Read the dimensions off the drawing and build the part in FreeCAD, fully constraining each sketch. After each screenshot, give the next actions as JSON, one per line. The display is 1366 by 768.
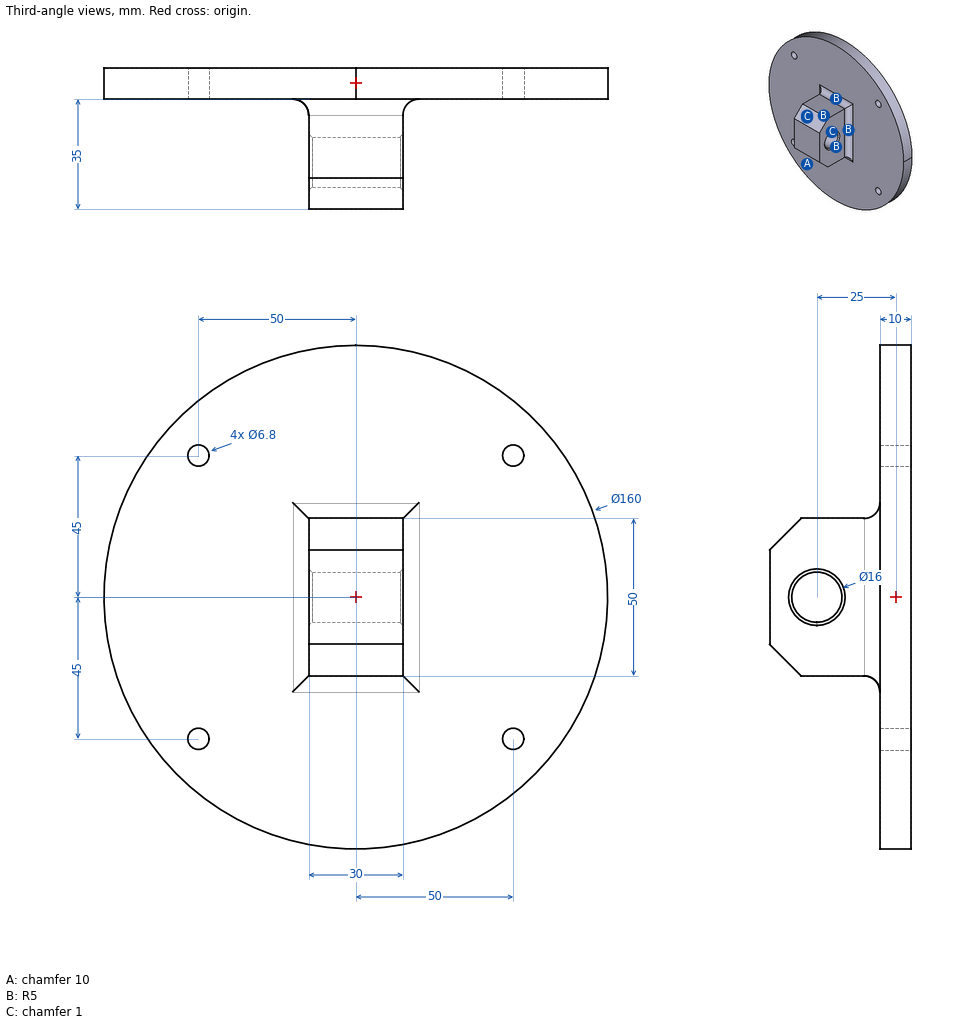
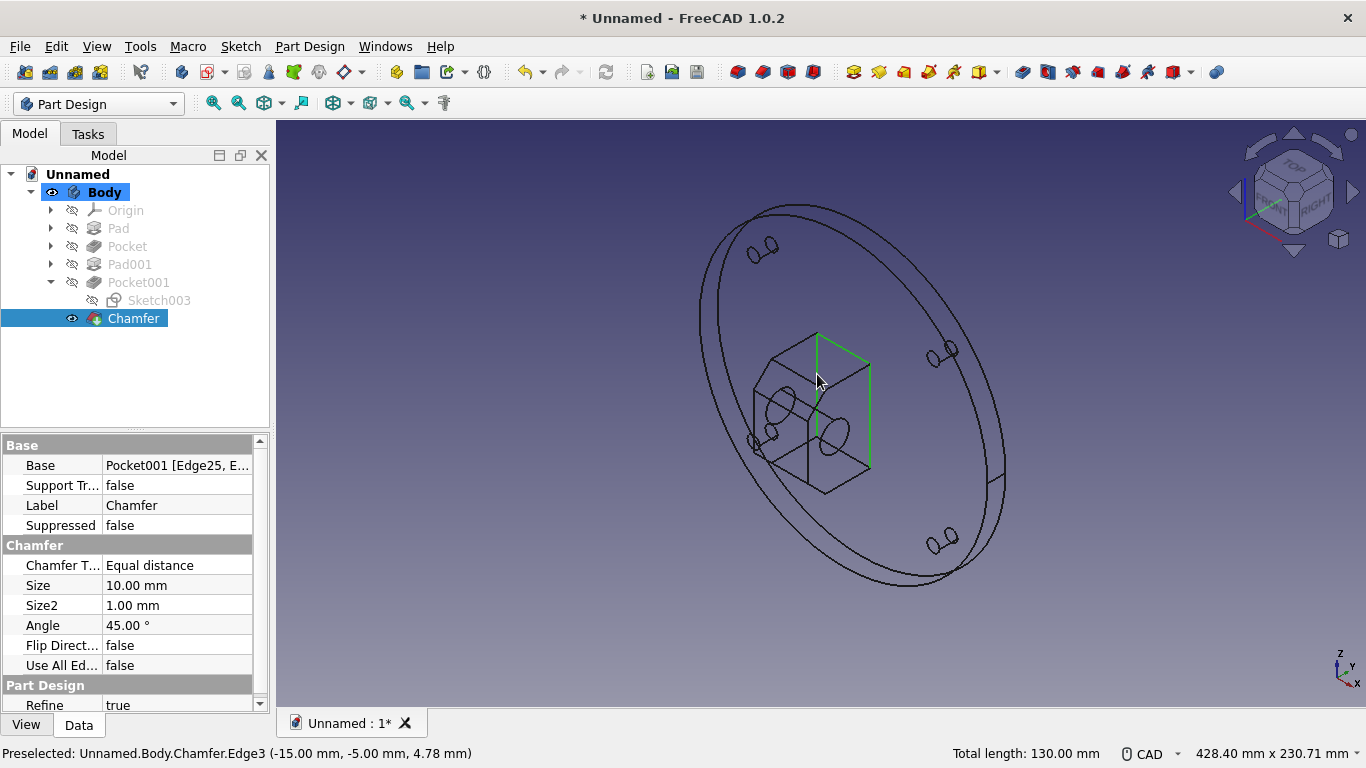
{"action": "left_click", "coordinate": [849, 455], "text": "ctrl"}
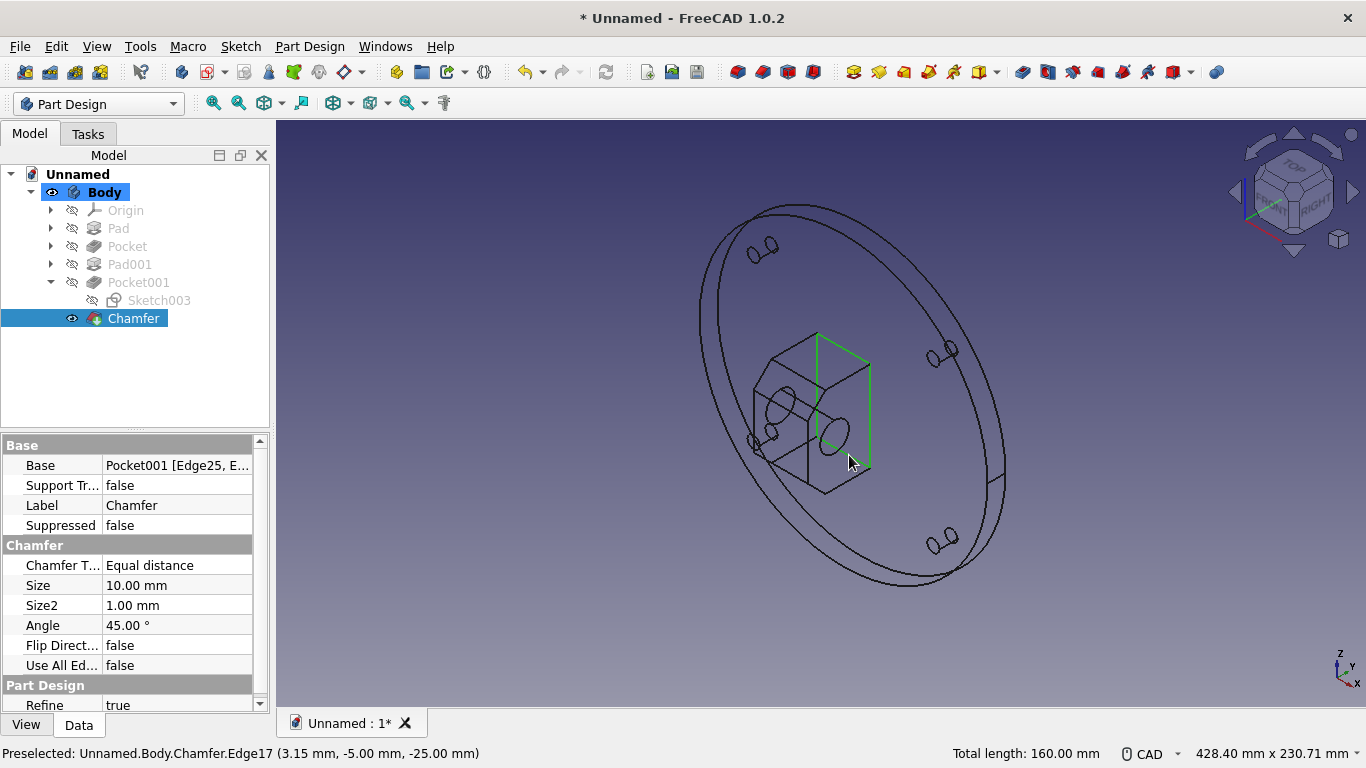
{"action": "key", "text": "v 1"}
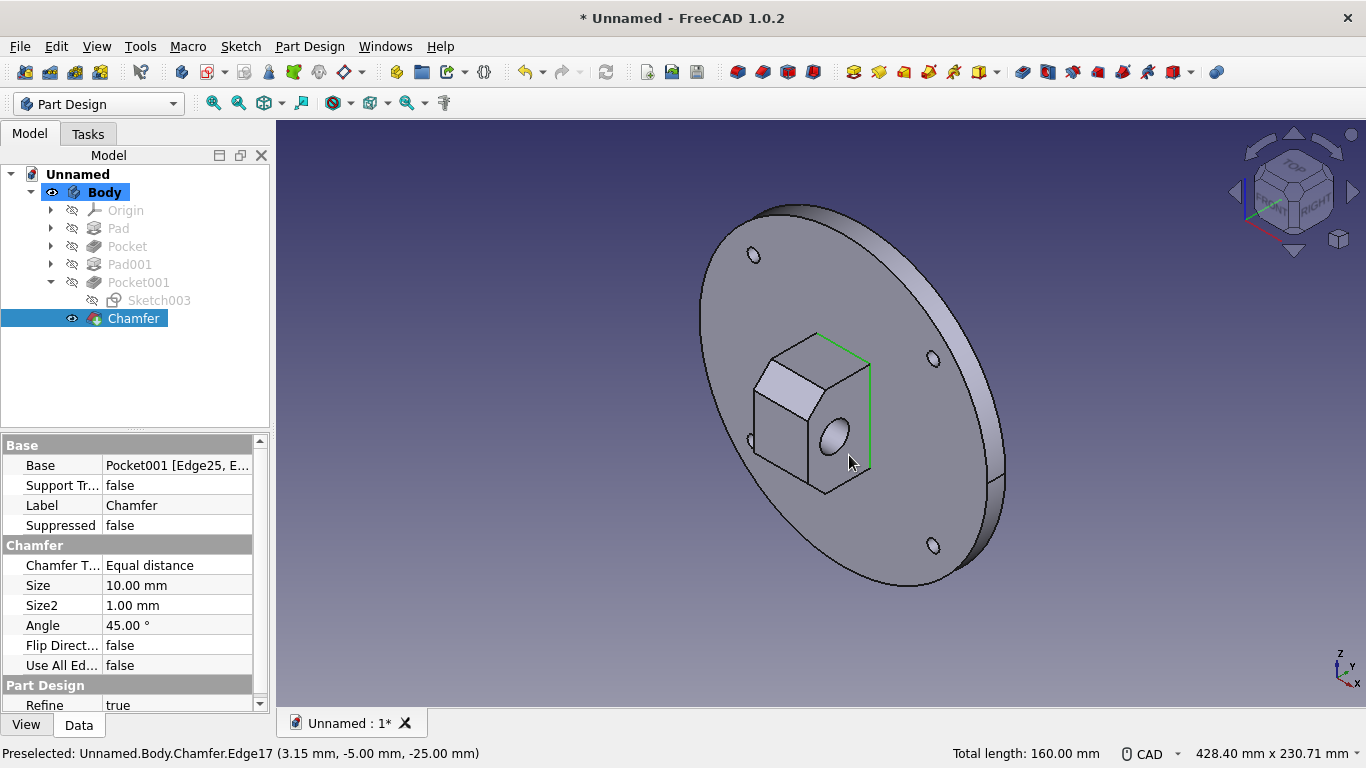
{"action": "left_click", "coordinate": [738, 72]}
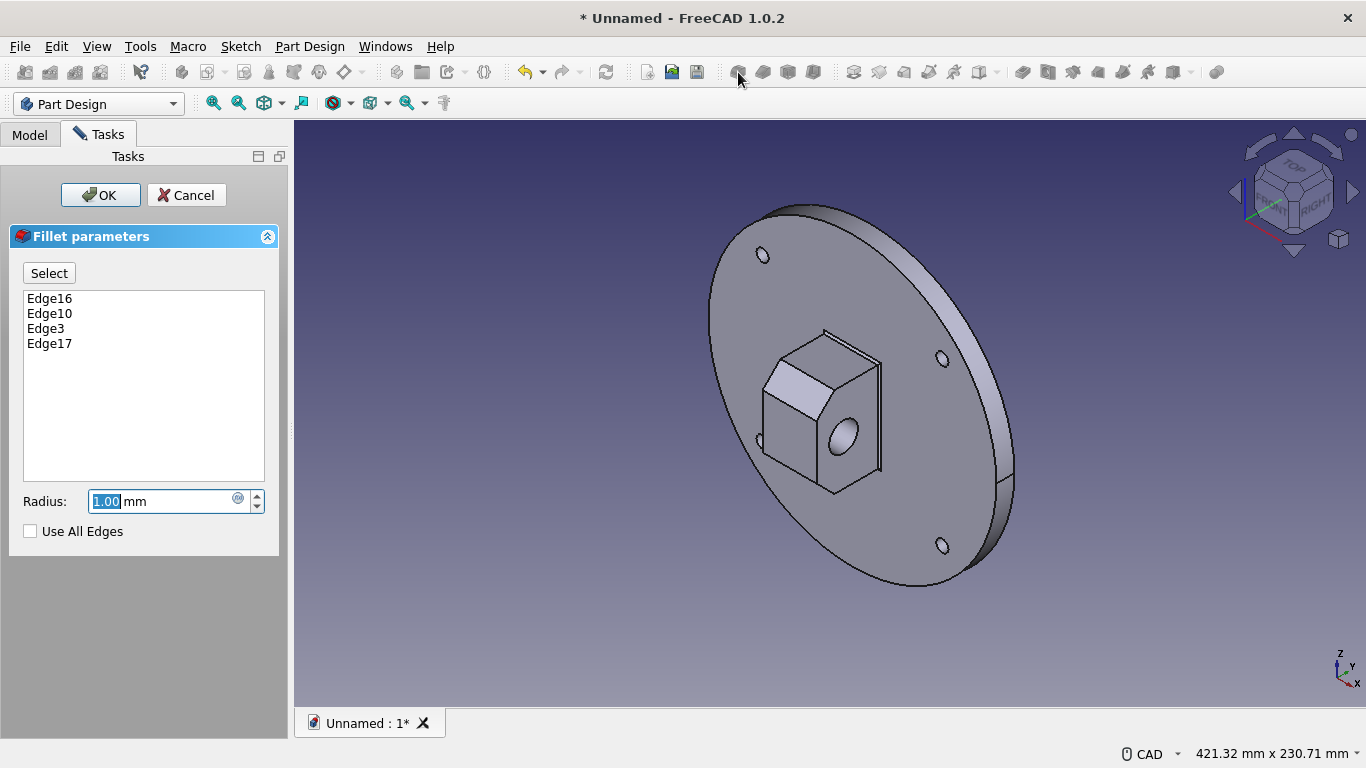
{"action": "type", "text": "5"}
{"action": "key", "text": "Tab"}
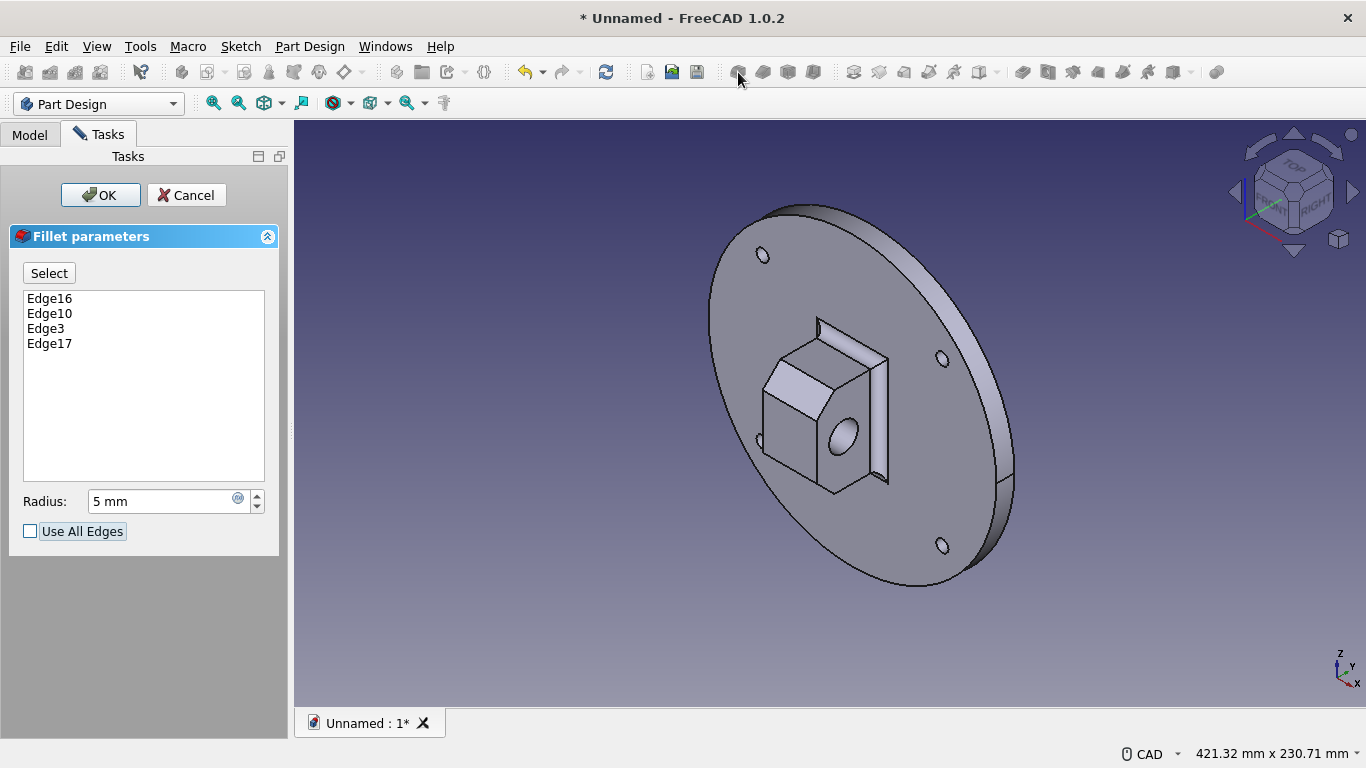
{"action": "left_click", "coordinate": [101, 195]}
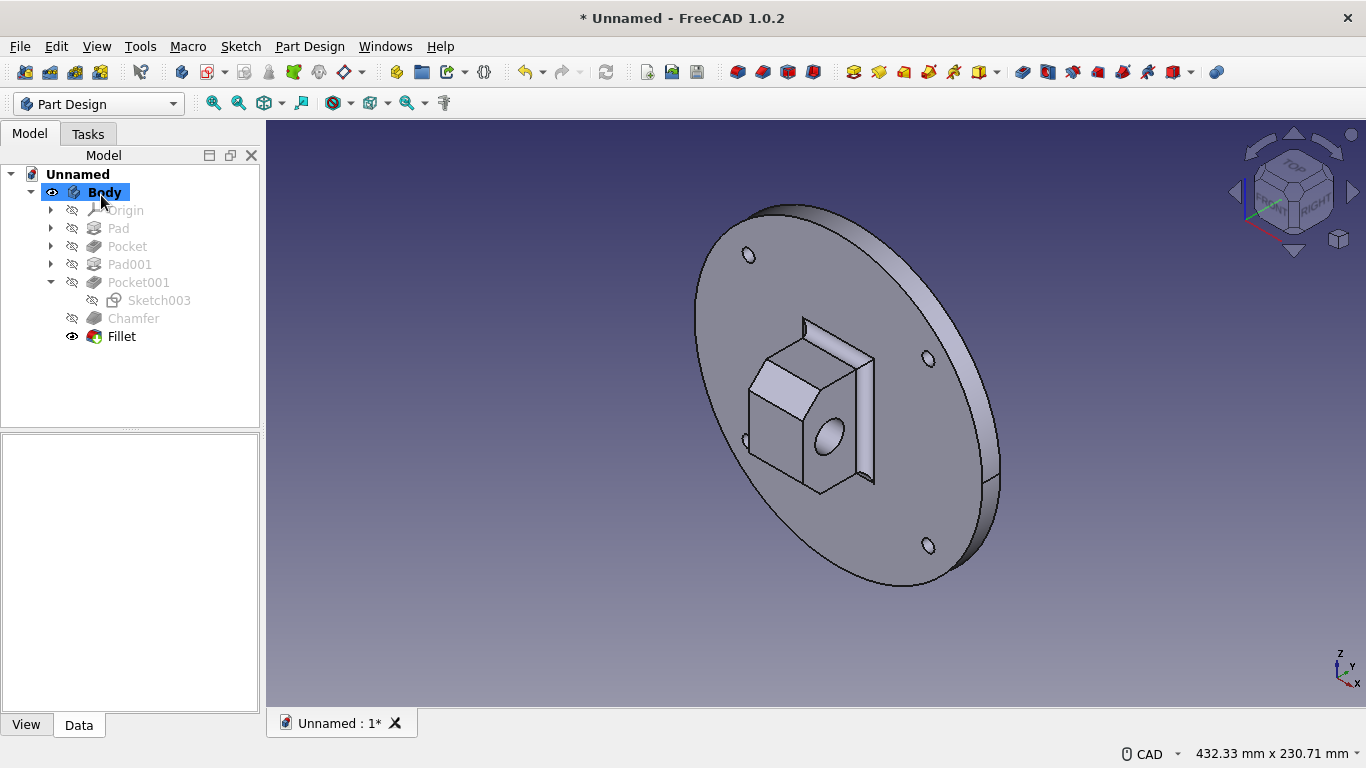
{"action": "left_click", "coordinate": [829, 452]}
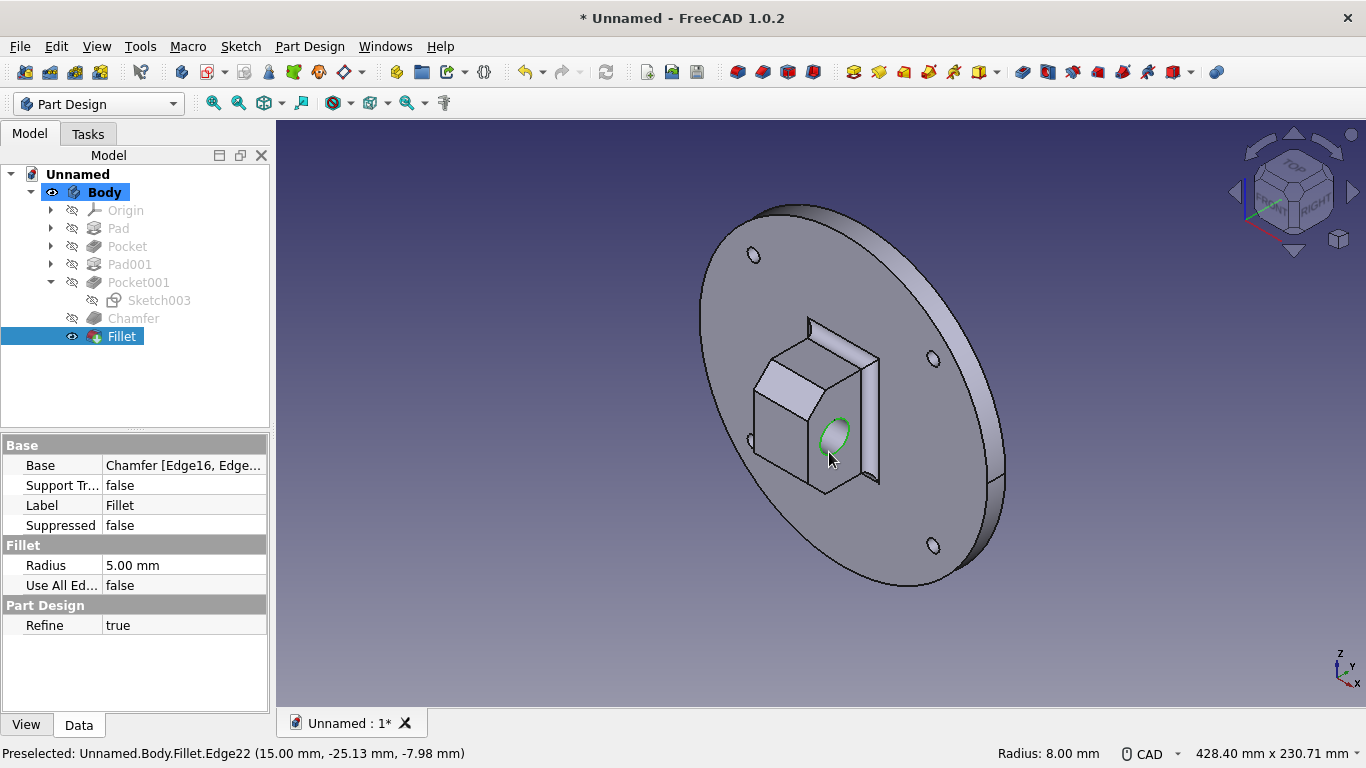
{"action": "key", "text": "2"}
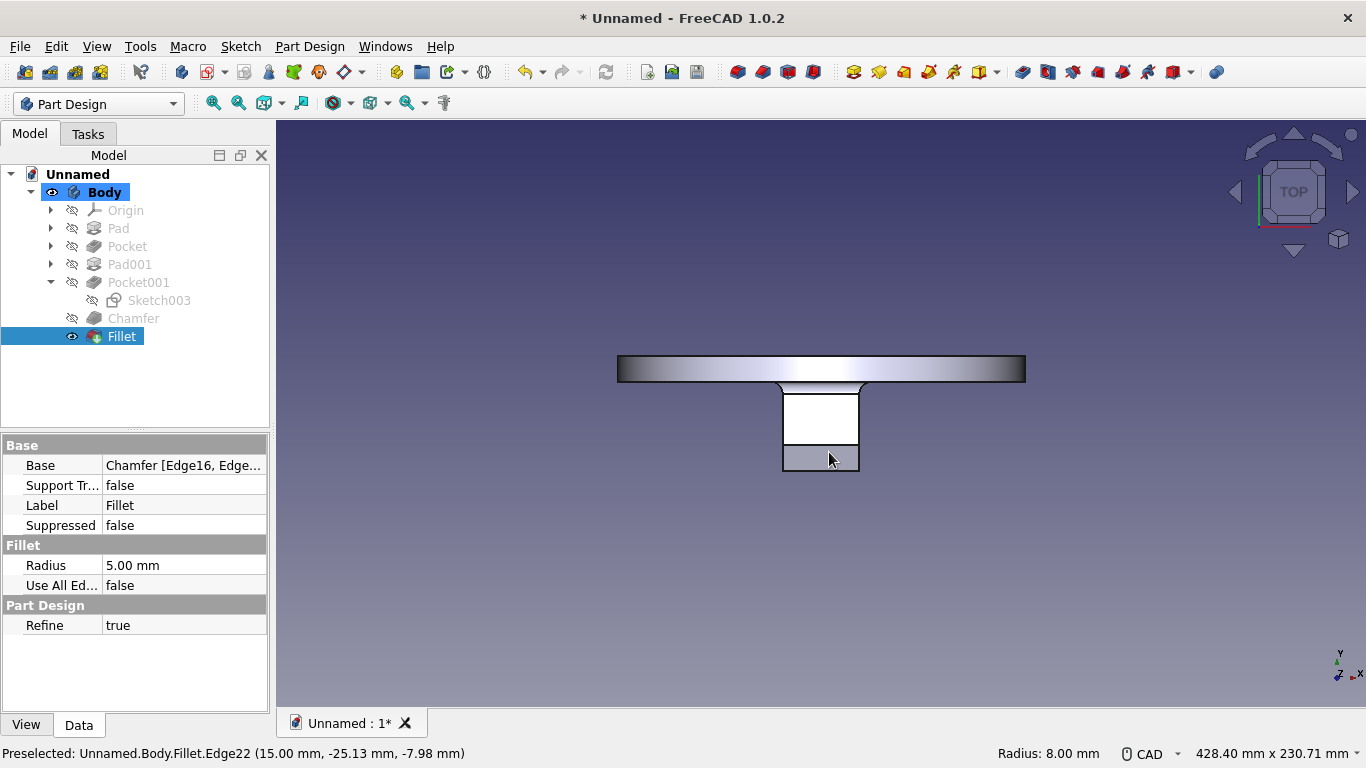
{"action": "left_click", "coordinate": [214, 104]}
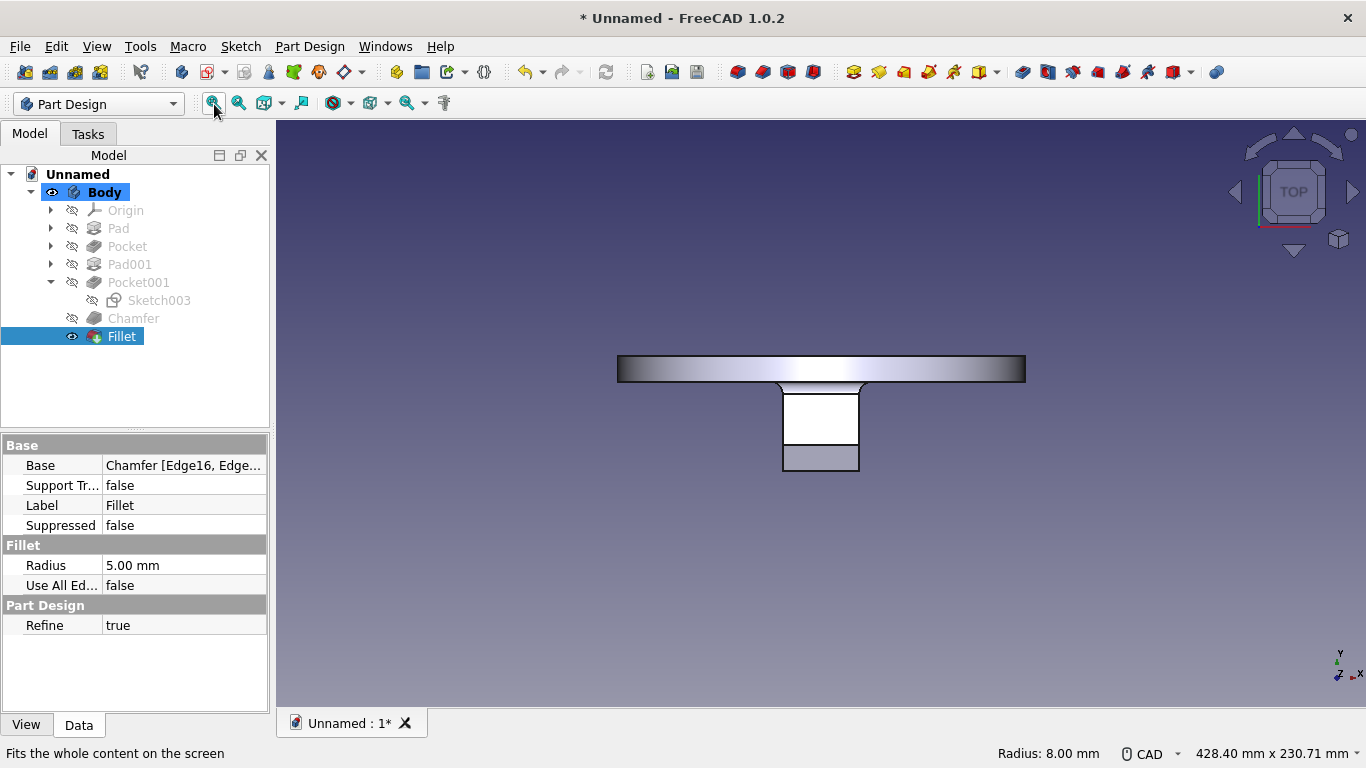
{"action": "key", "text": "0"}